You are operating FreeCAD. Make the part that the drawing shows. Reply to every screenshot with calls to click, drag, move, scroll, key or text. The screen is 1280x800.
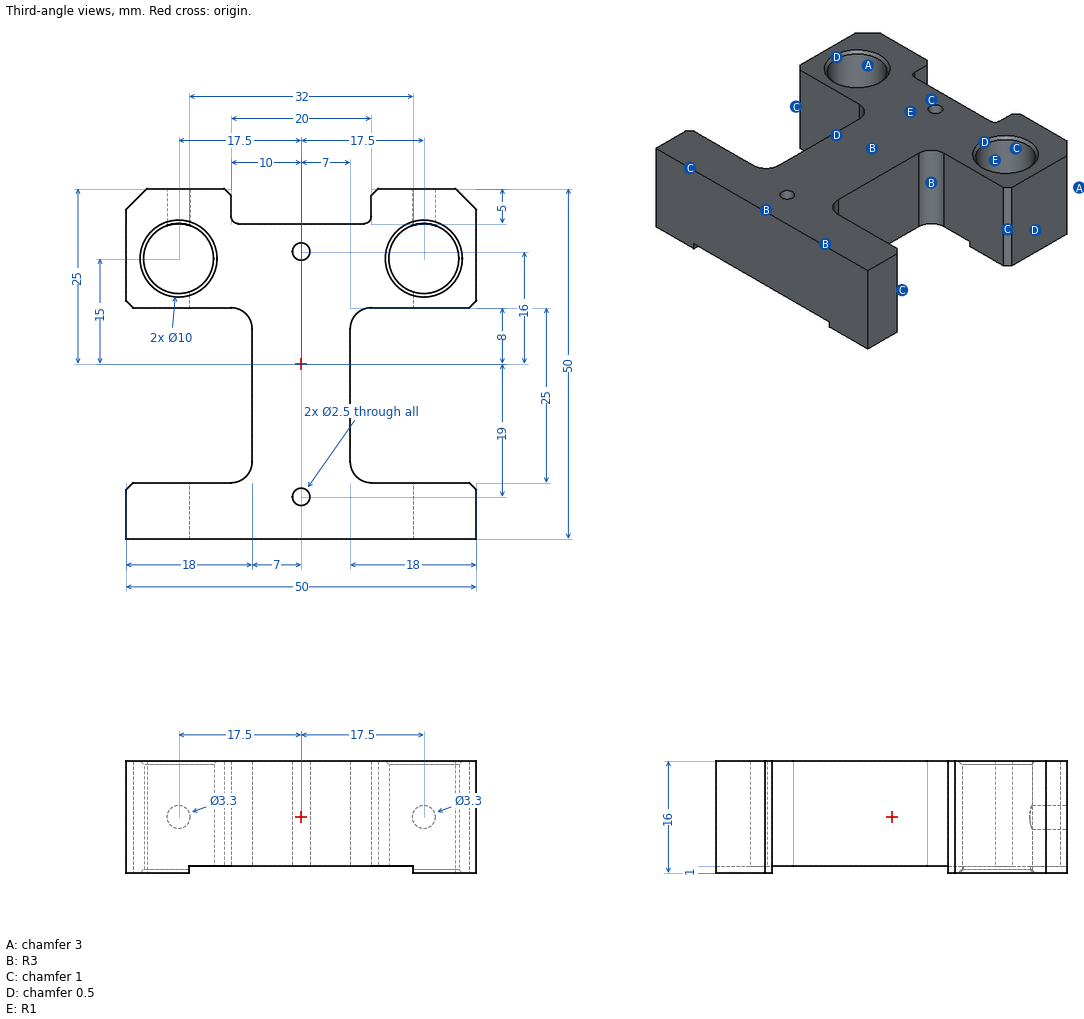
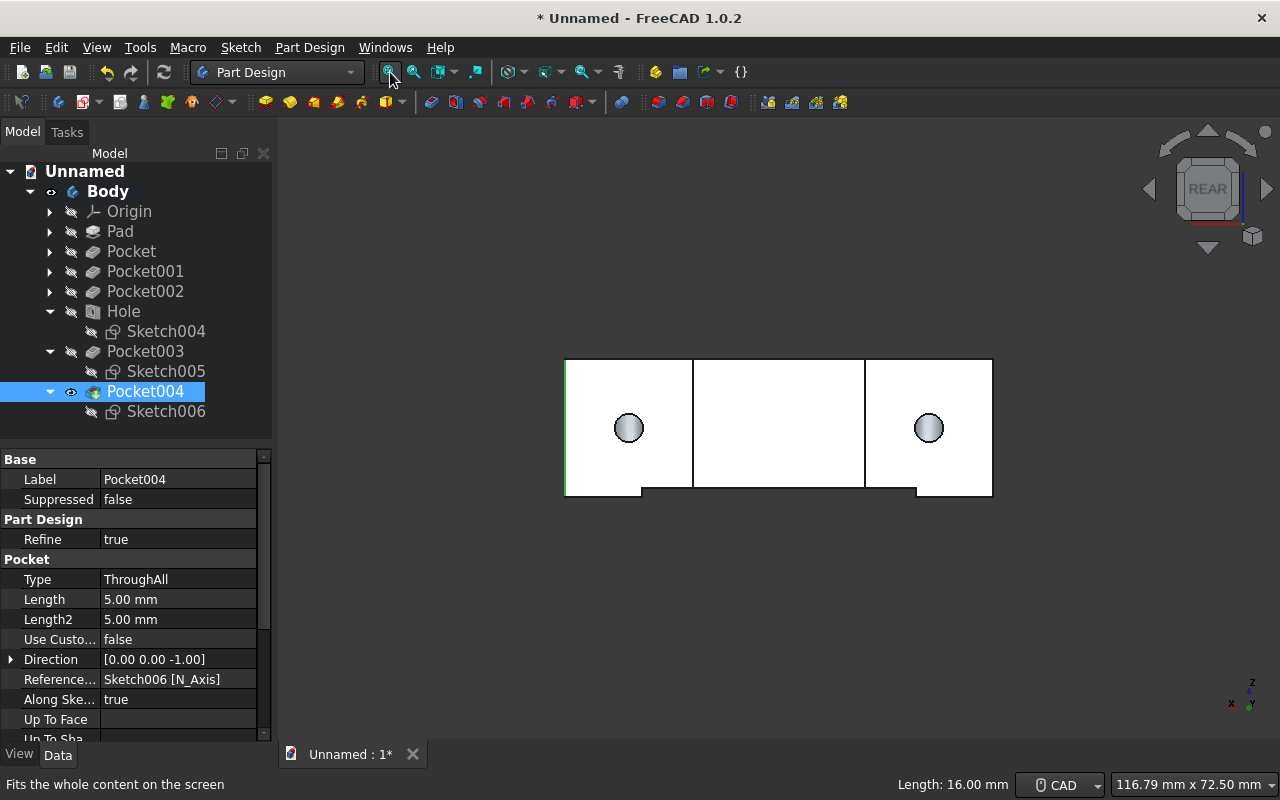
click(993, 427, ctrl)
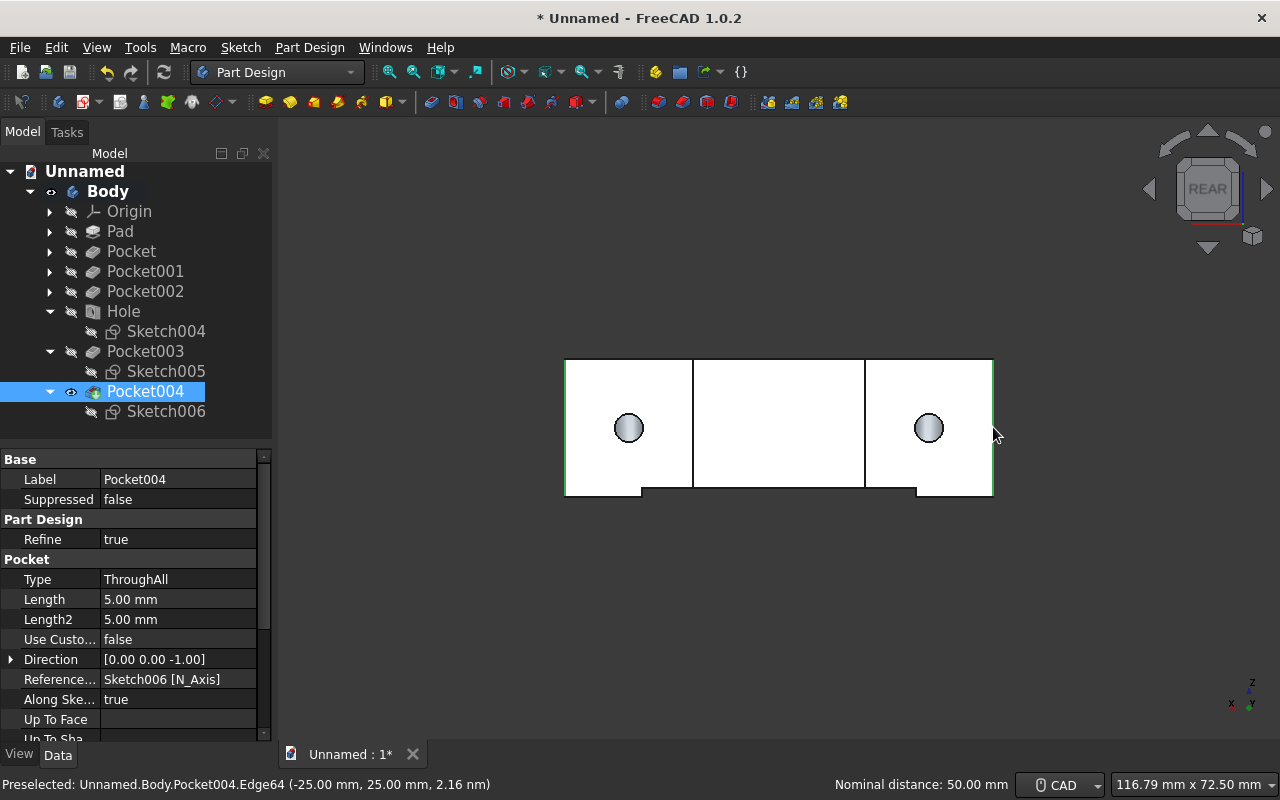
click(684, 102)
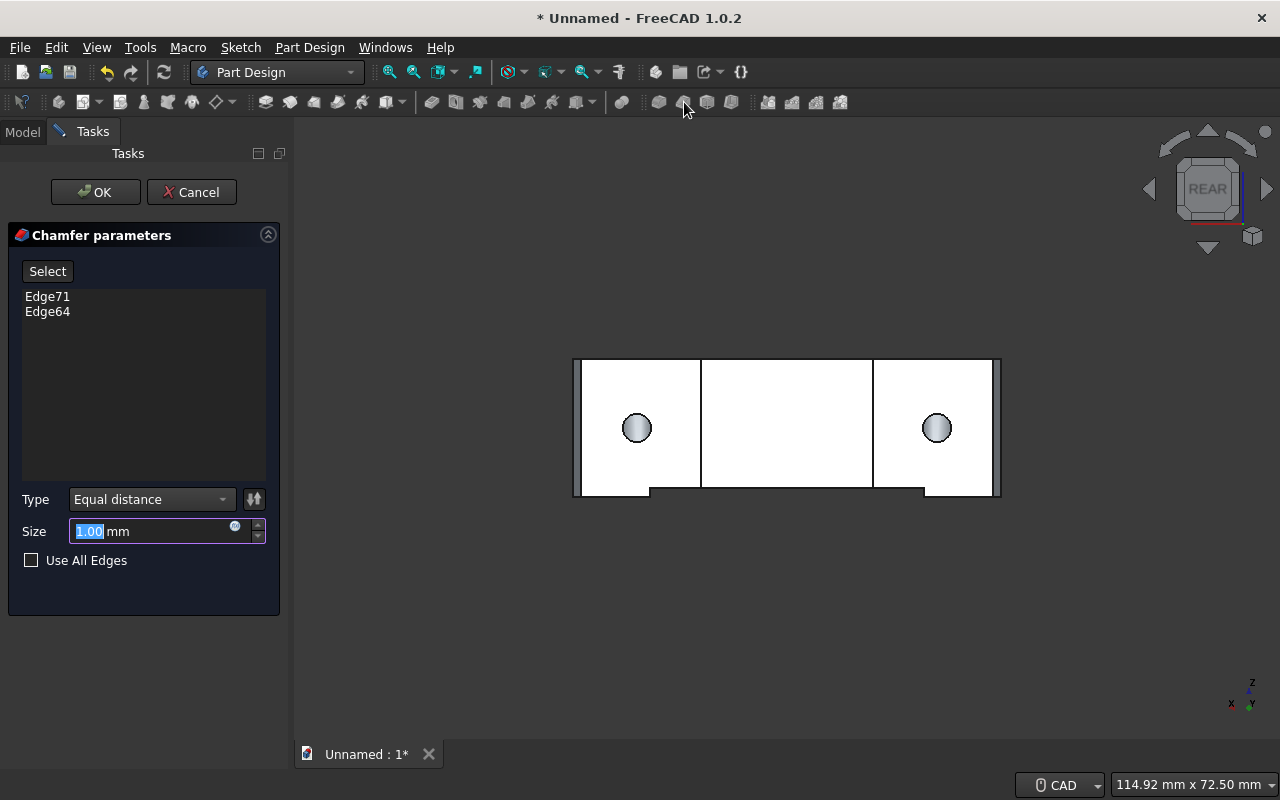
text(3)
key(Tab)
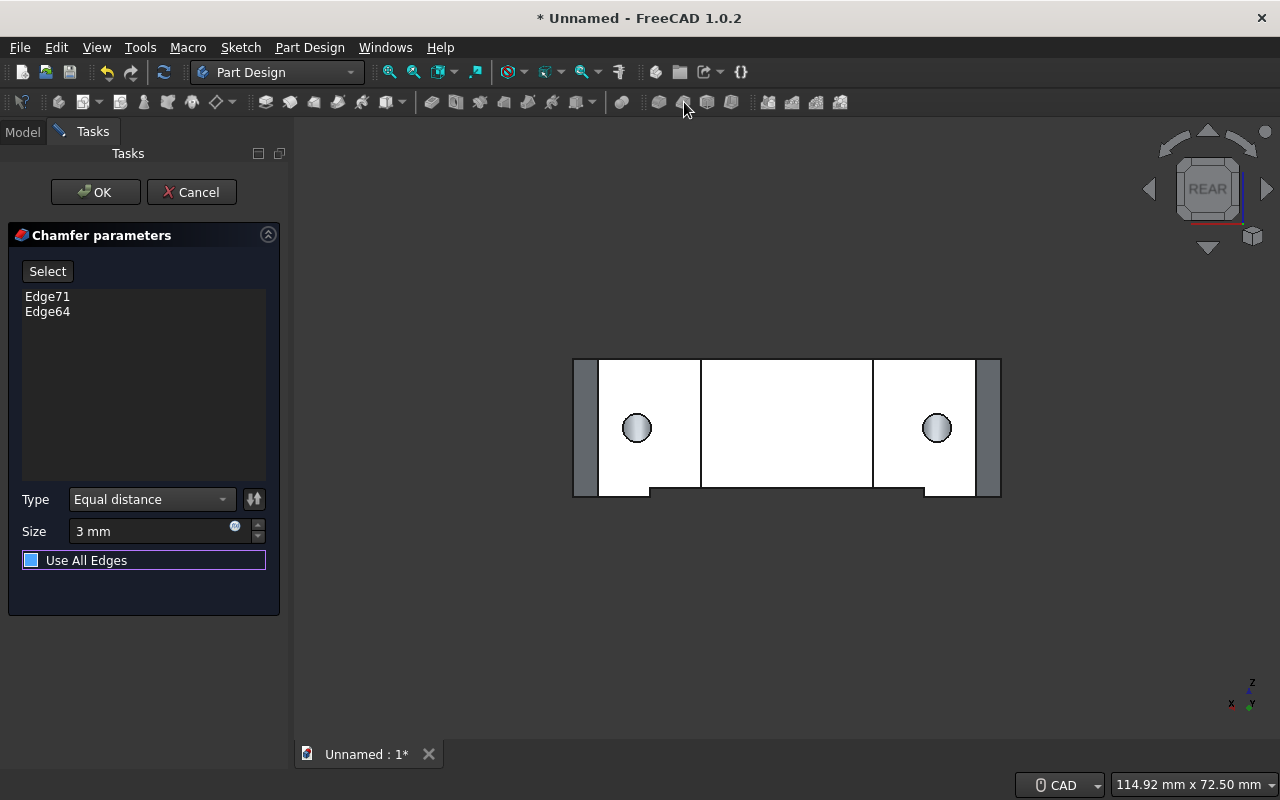
click(96, 192)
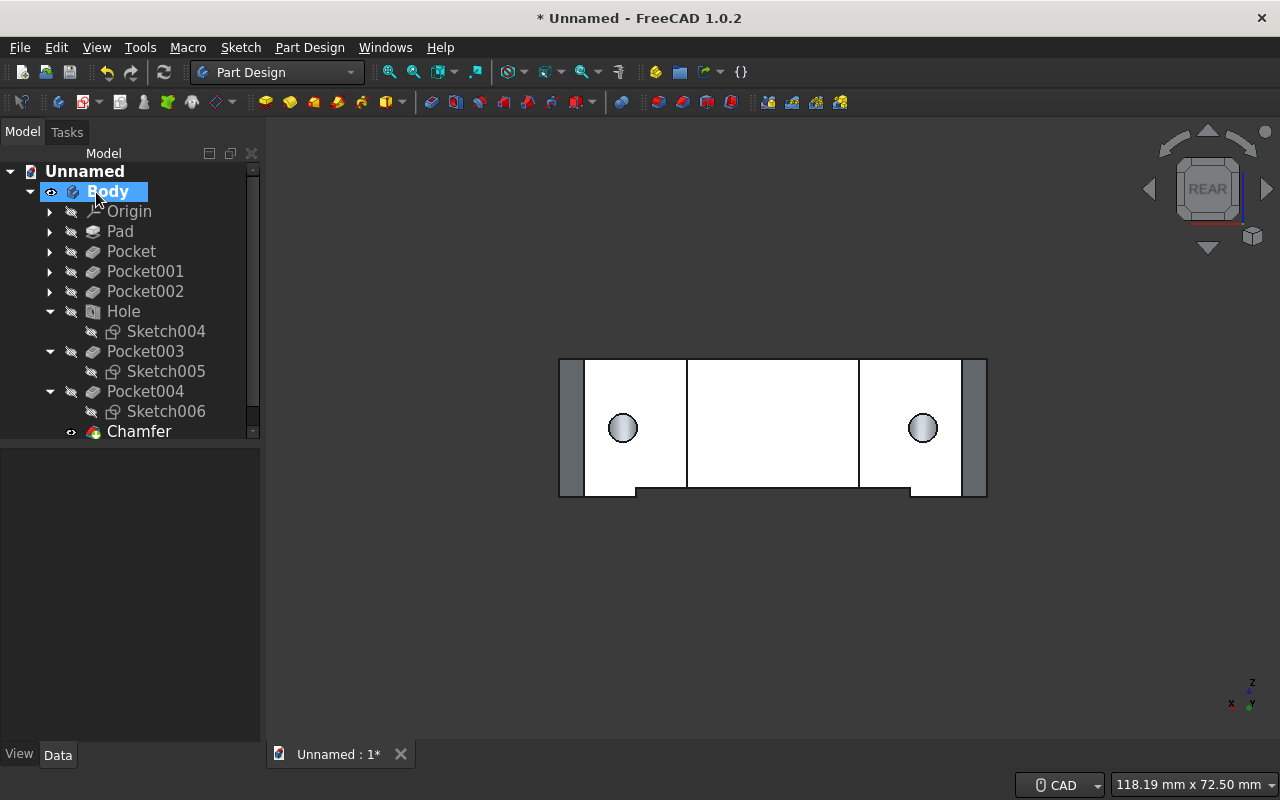
key(v)
key(f)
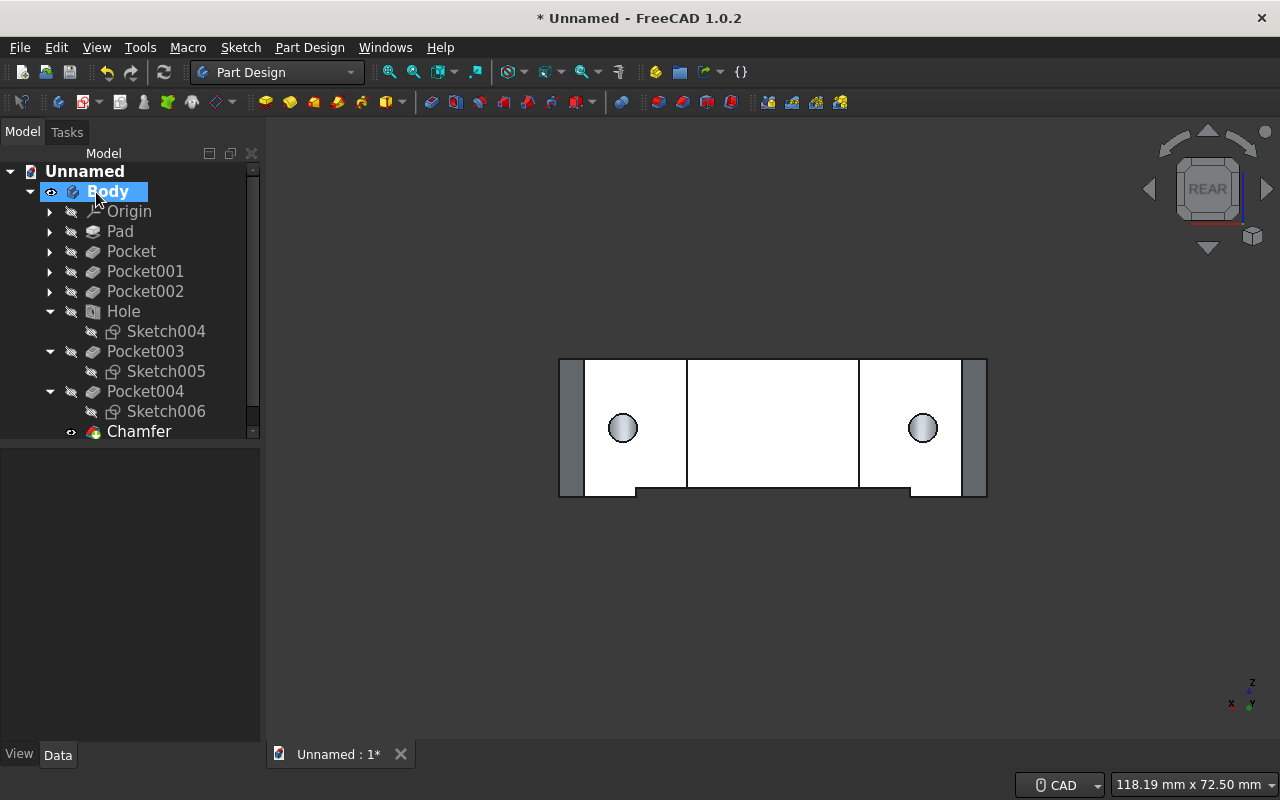
key(0)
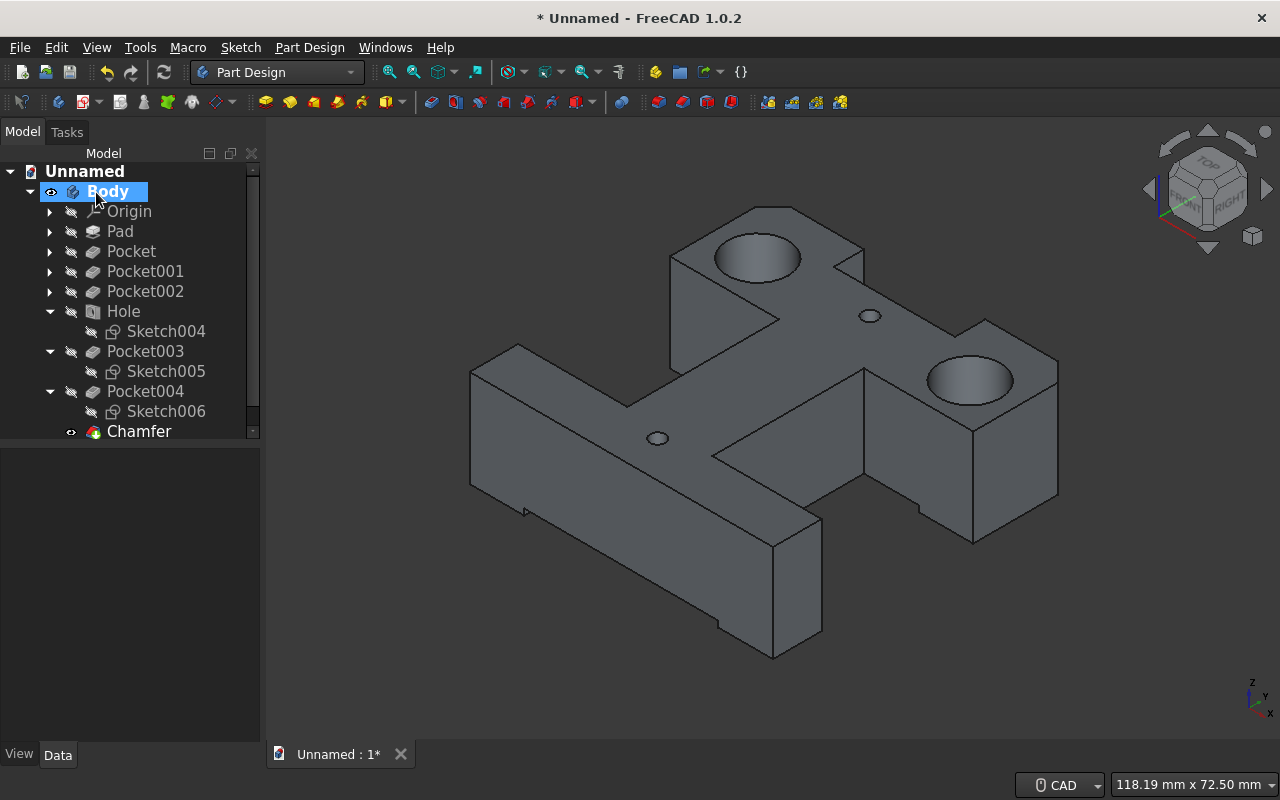
key(2)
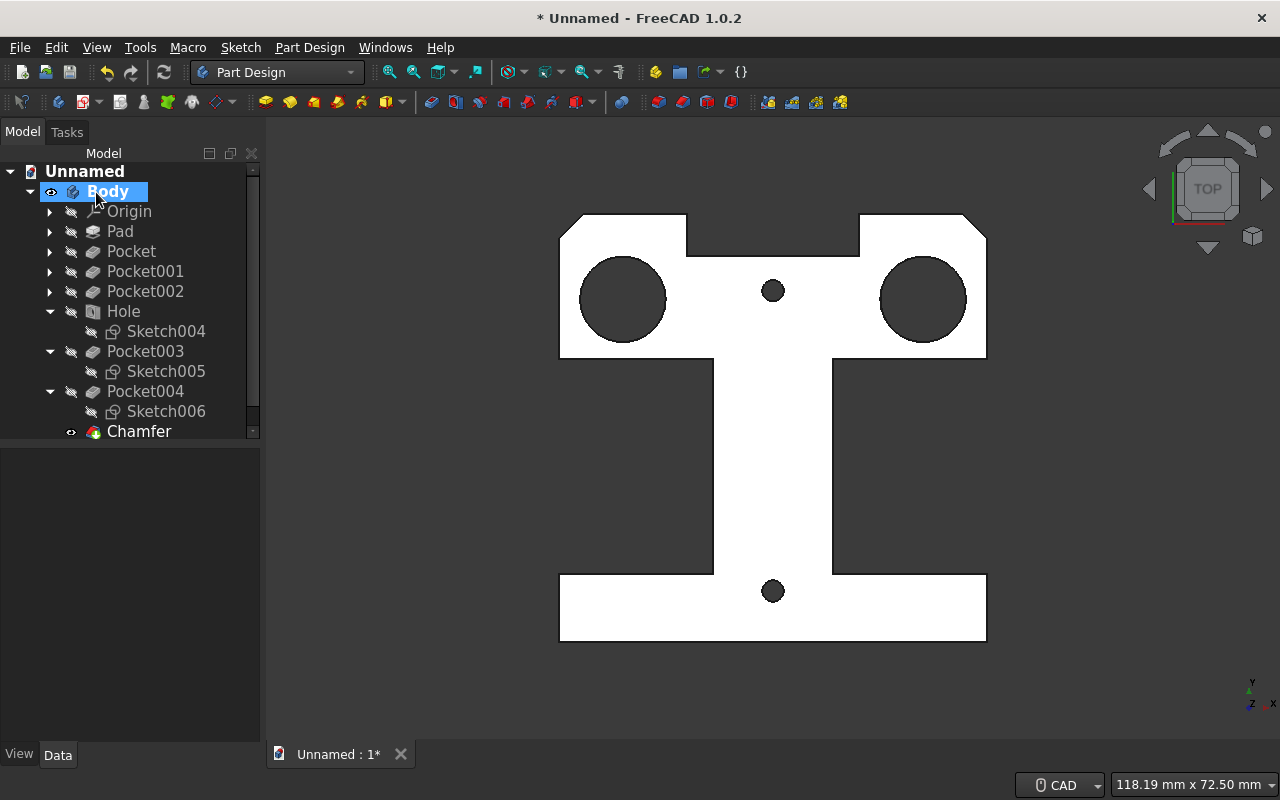
key(1)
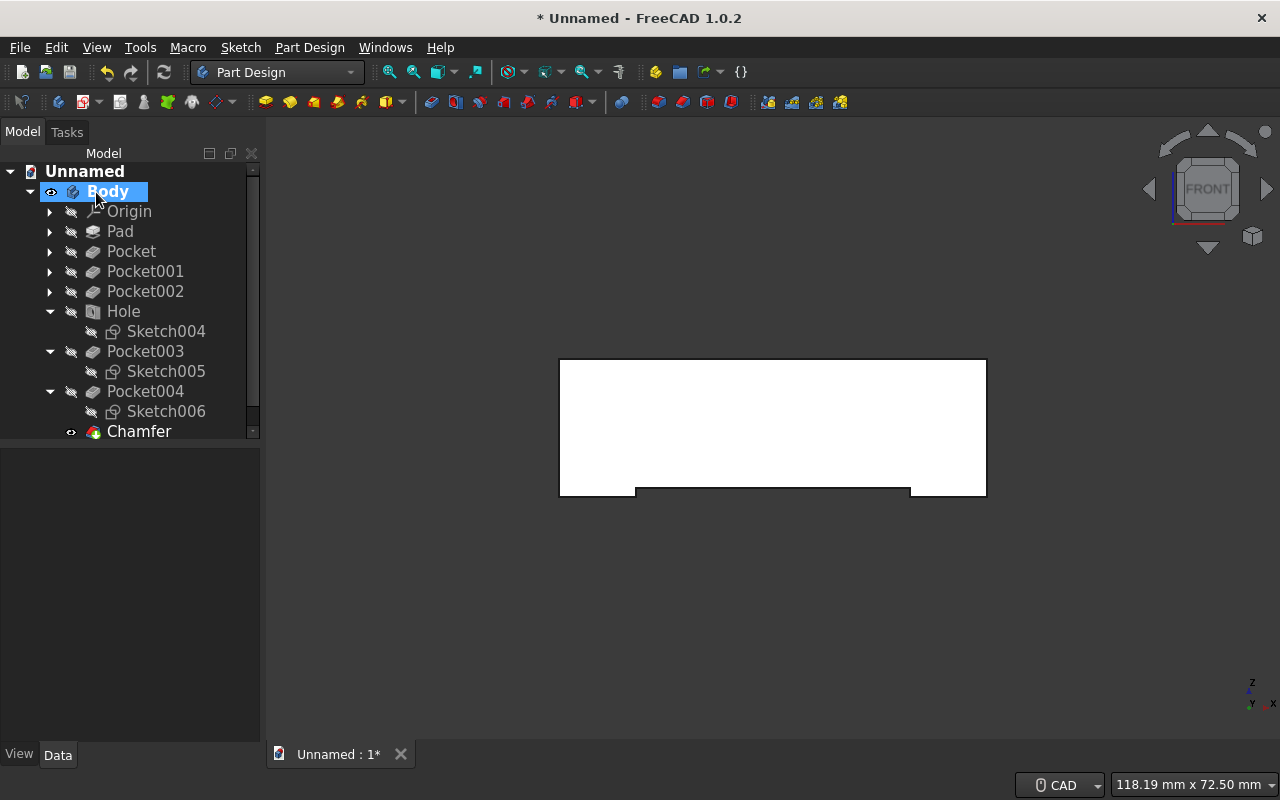
key(v)
key(f)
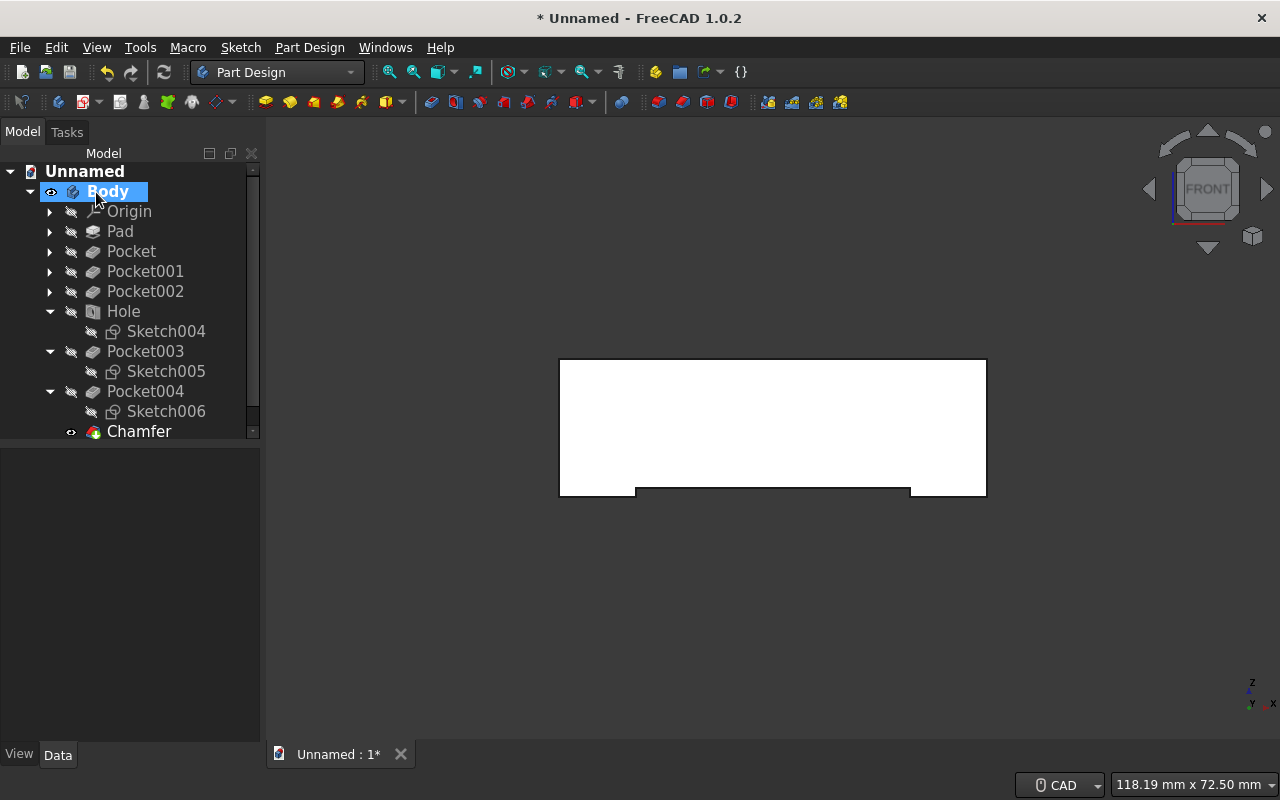
key(3)